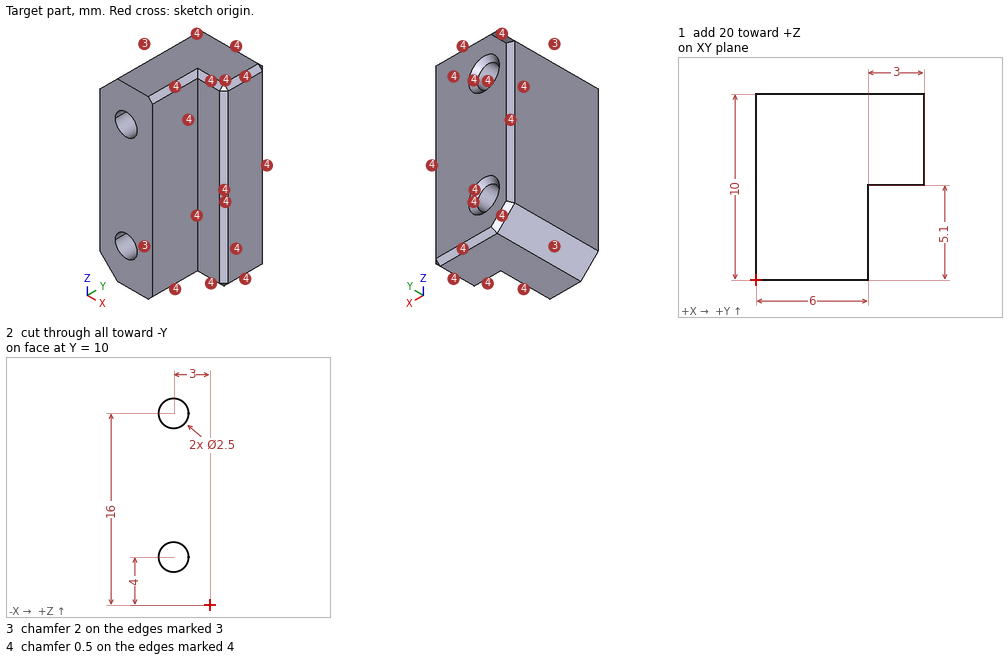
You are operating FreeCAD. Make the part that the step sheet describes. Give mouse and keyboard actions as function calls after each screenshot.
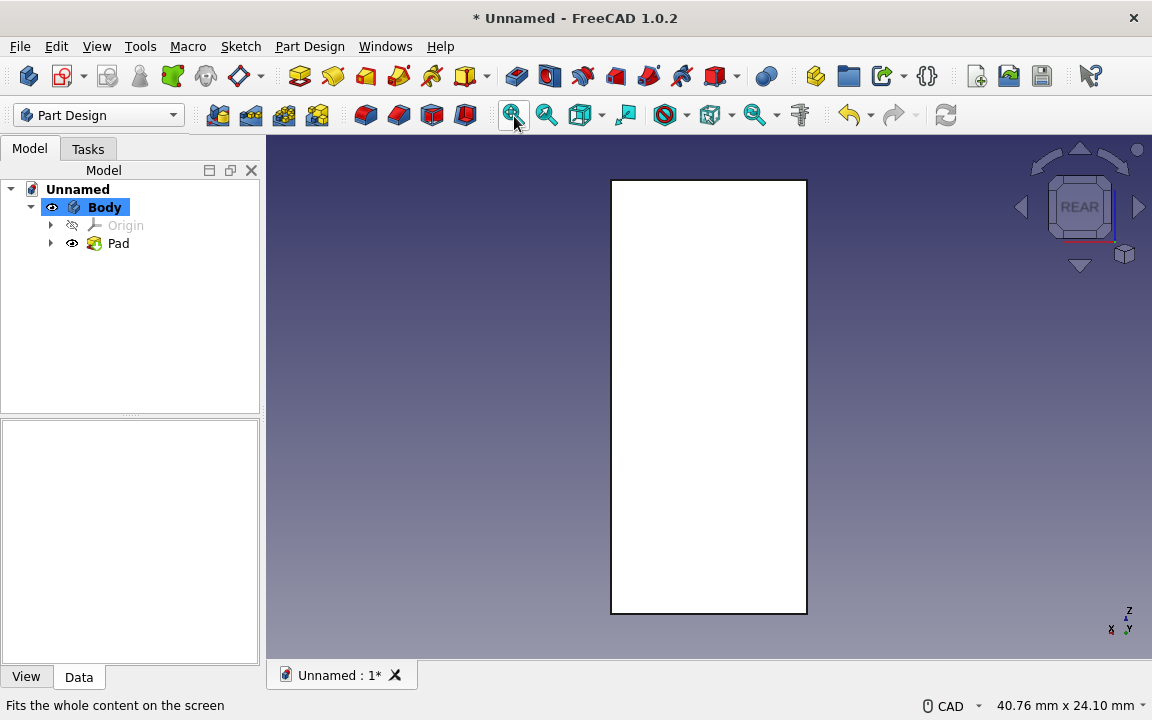
click(709, 334)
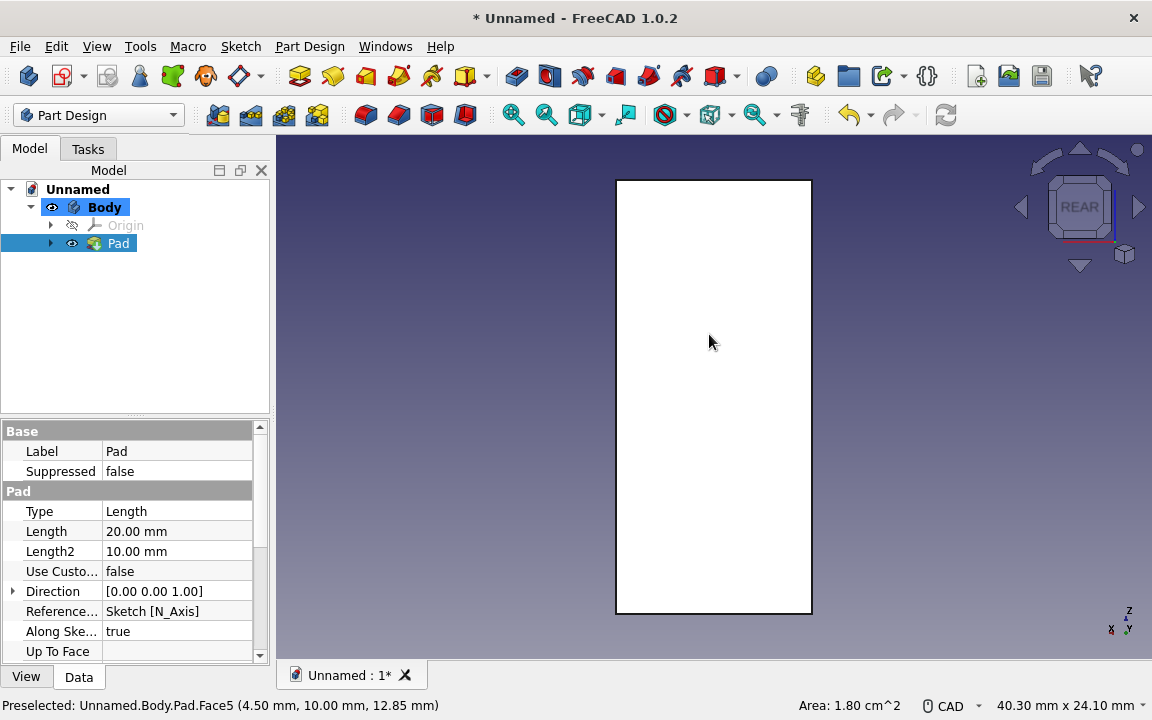
click(62, 76)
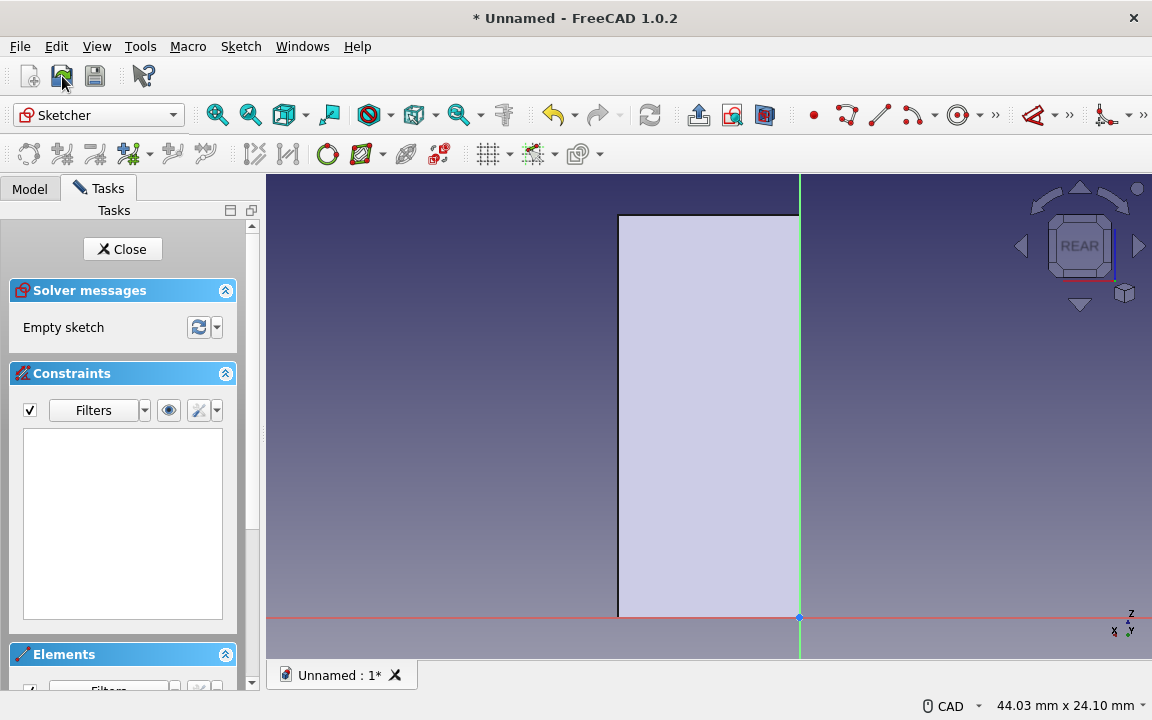
scroll(294, 292, down, 1)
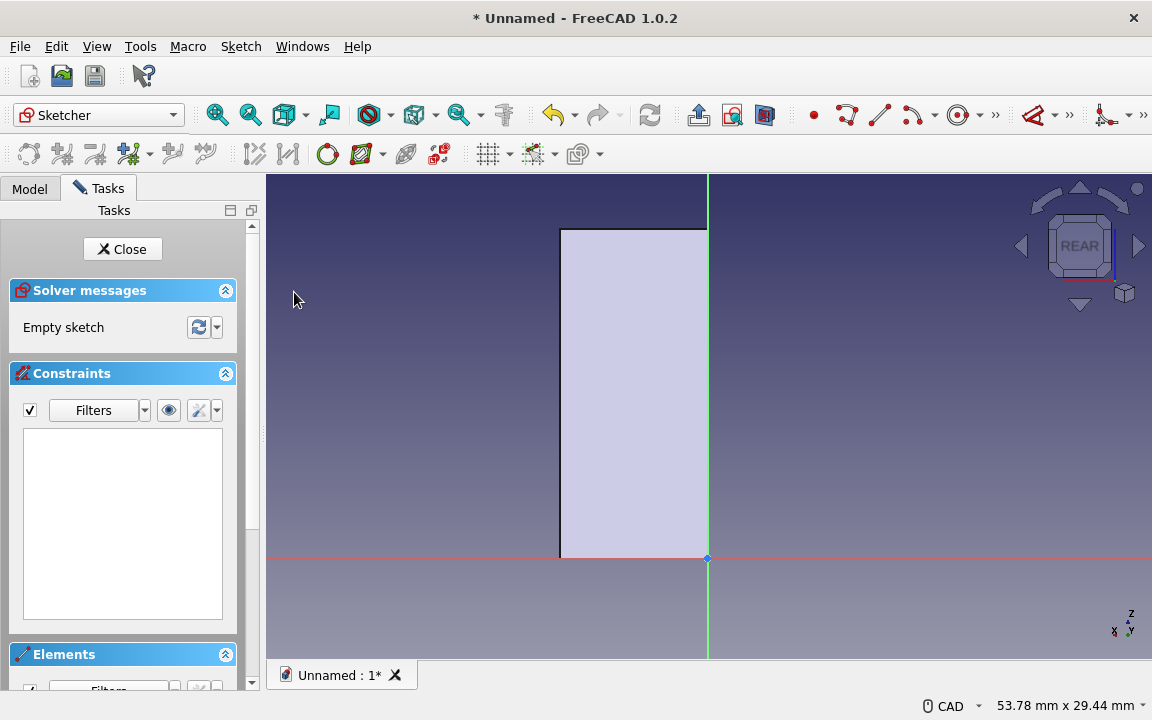
click(958, 116)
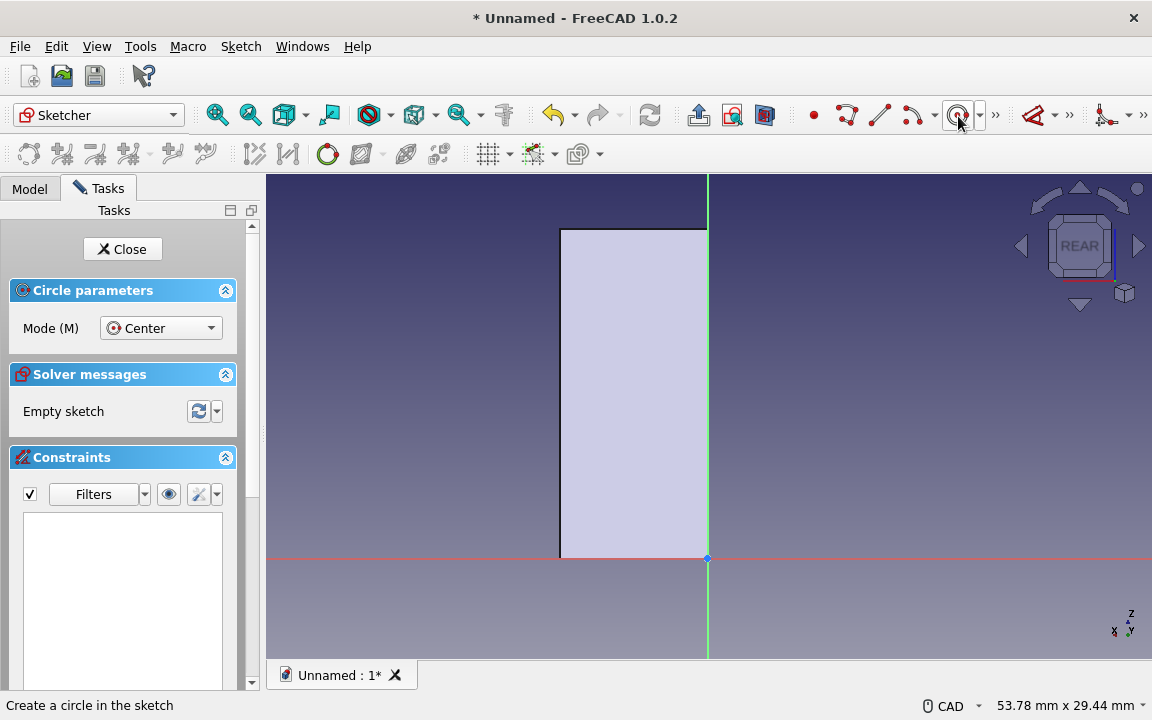
click(658, 295)
move(673, 281)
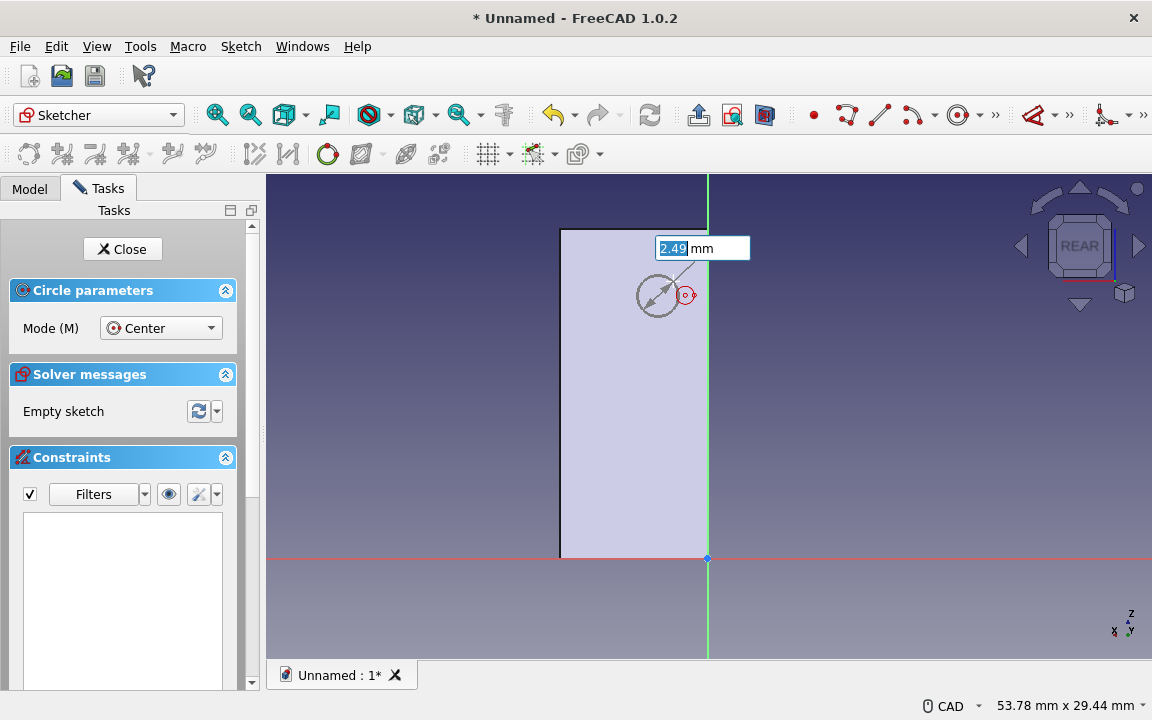
text(2.5)
key(Return)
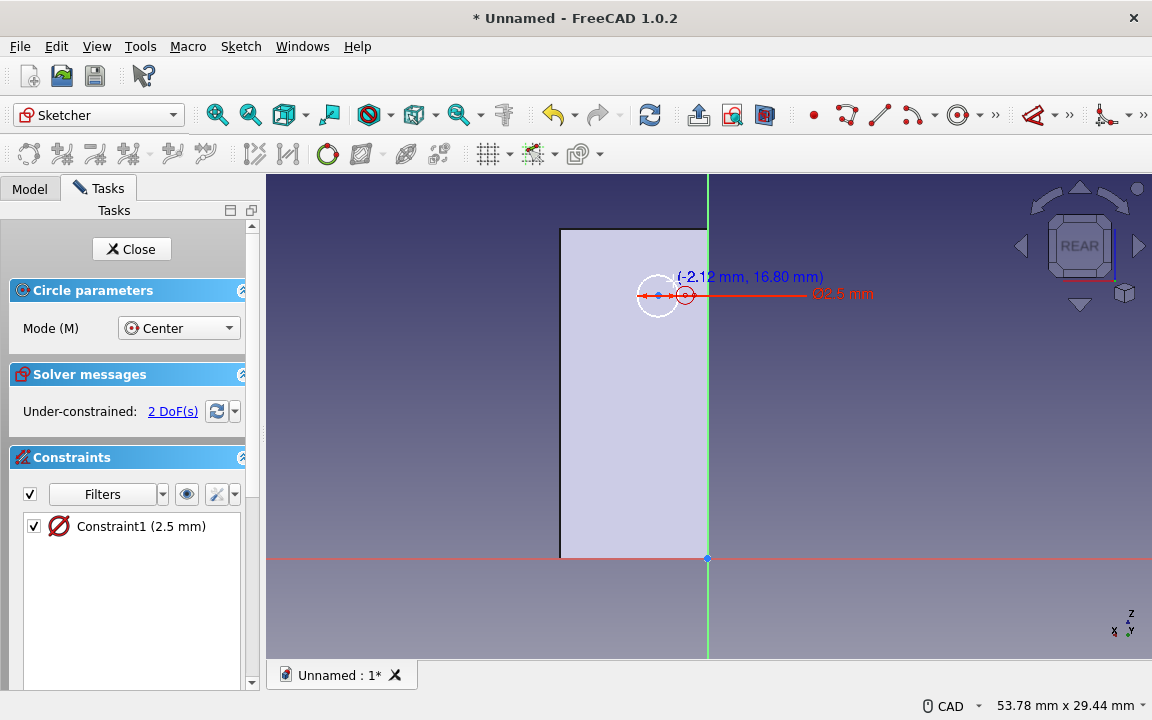
click(658, 493)
move(673, 478)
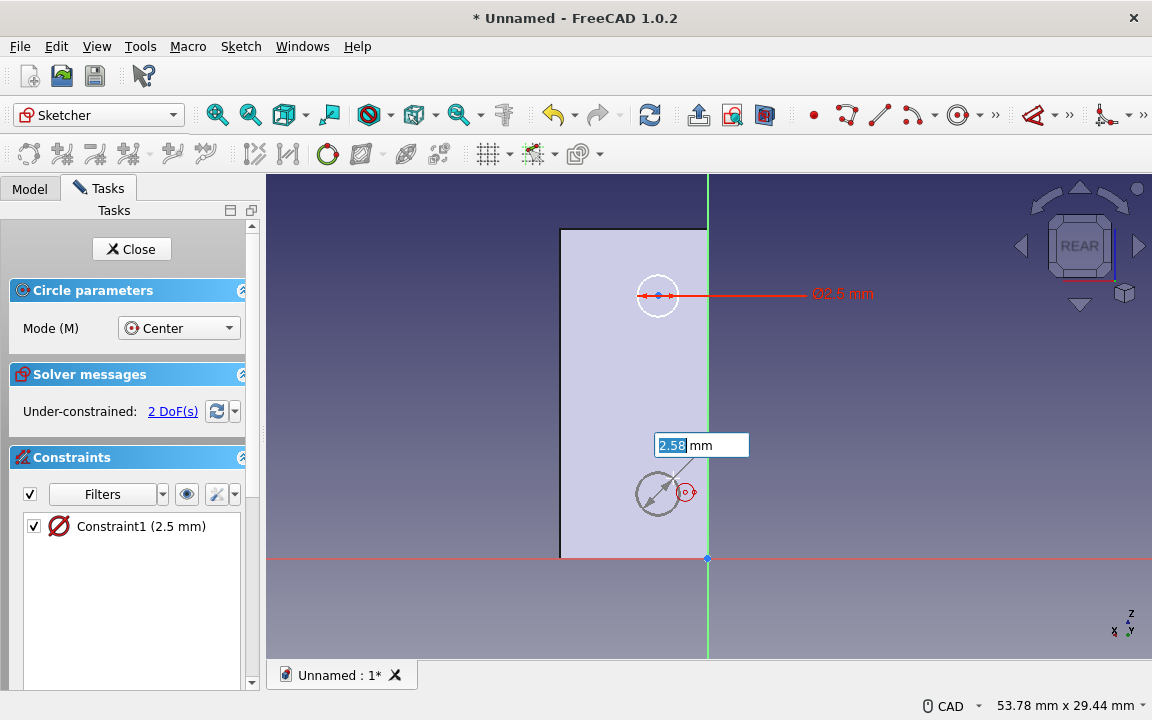
text(2.5)
key(Return)
key(Escape)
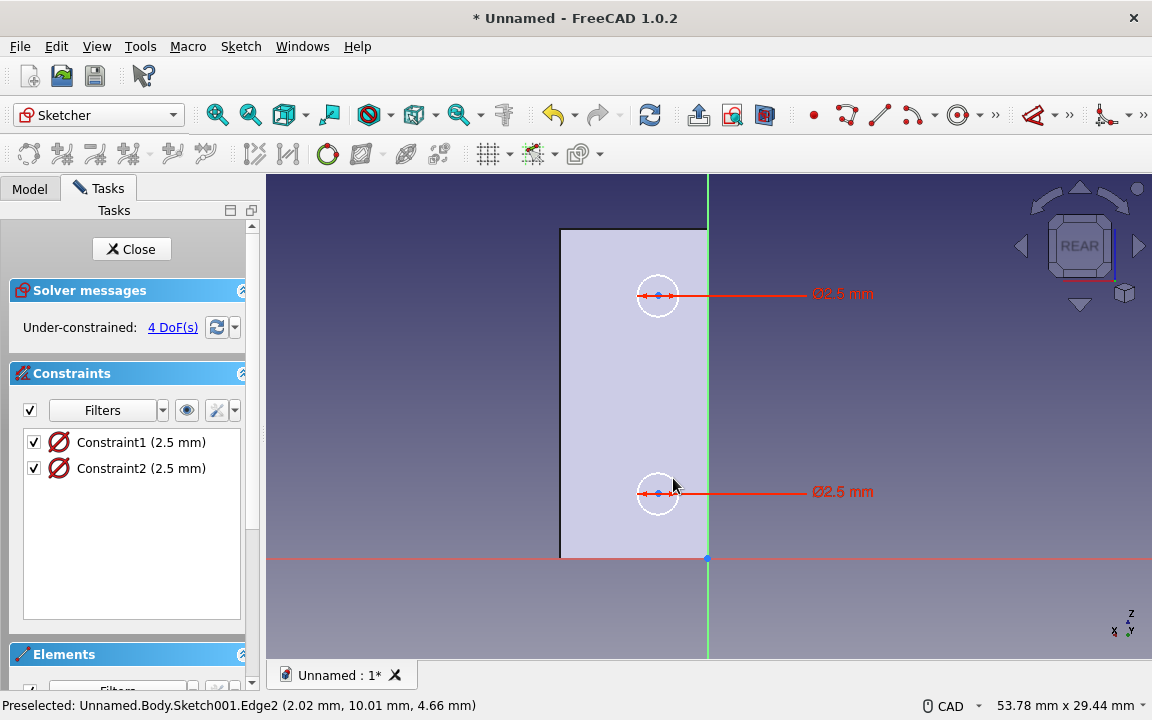
click(658, 296)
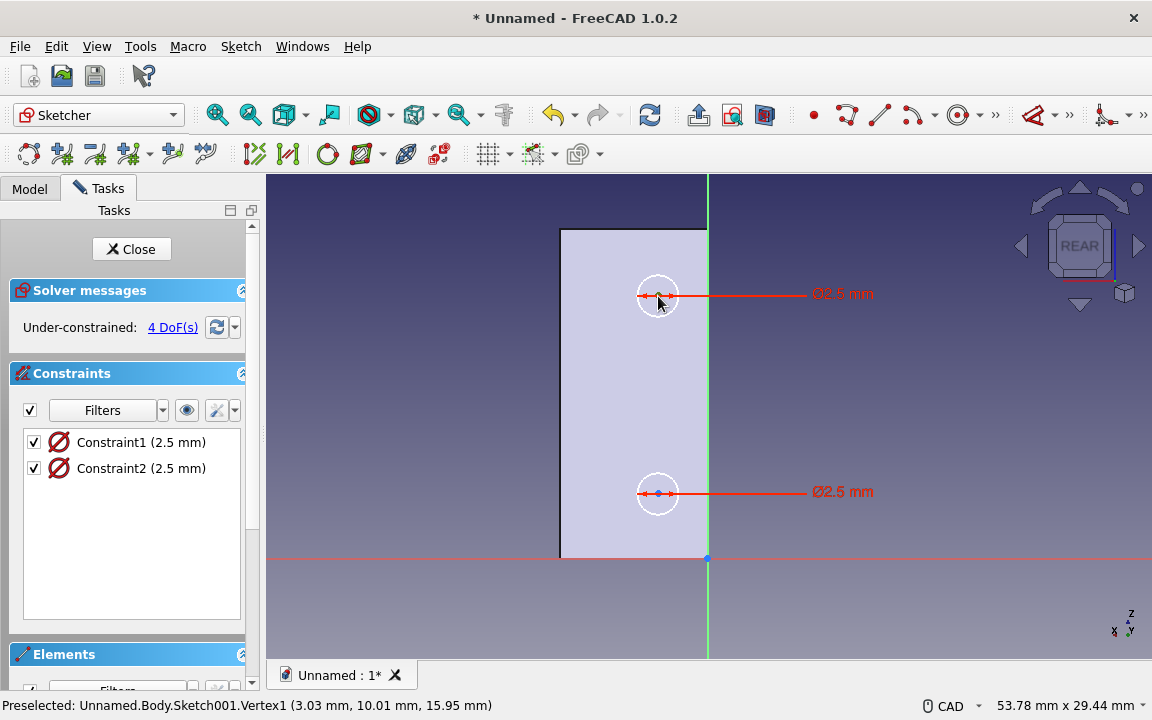
click(658, 494)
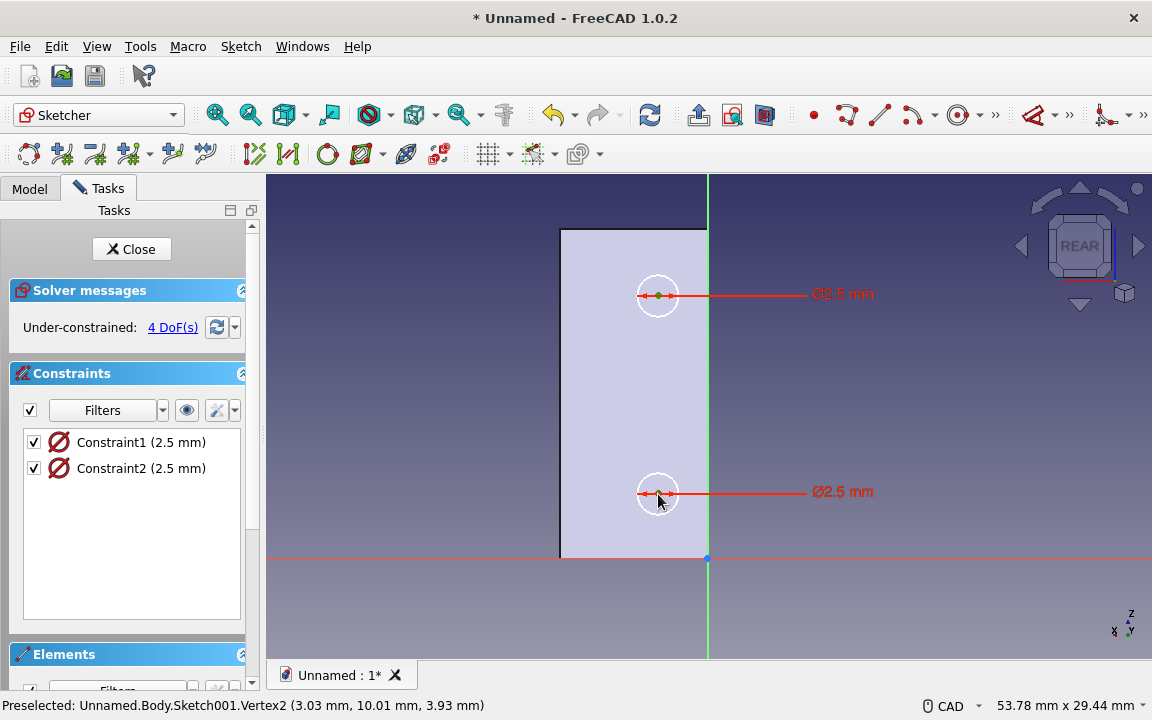
key(v)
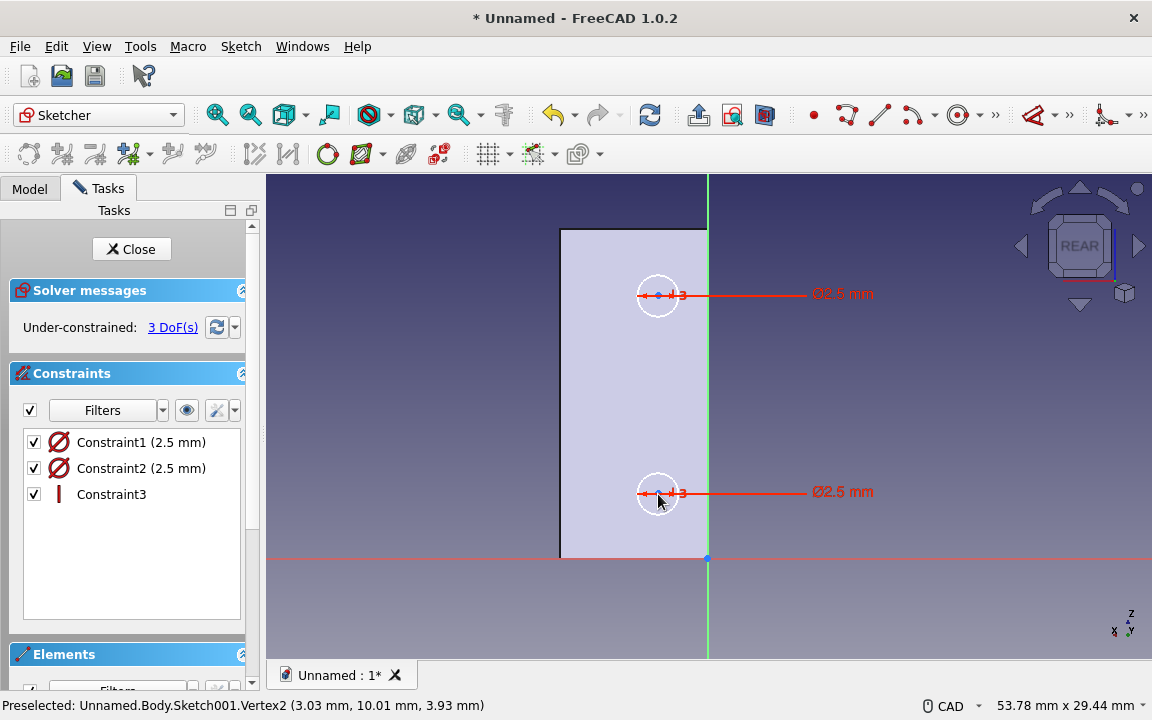
click(1032, 116)